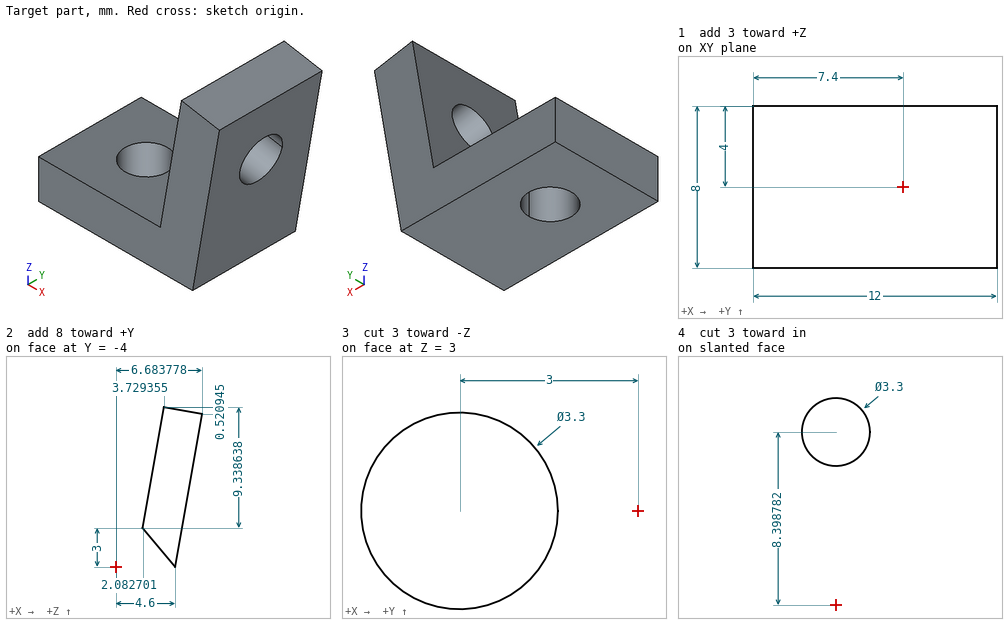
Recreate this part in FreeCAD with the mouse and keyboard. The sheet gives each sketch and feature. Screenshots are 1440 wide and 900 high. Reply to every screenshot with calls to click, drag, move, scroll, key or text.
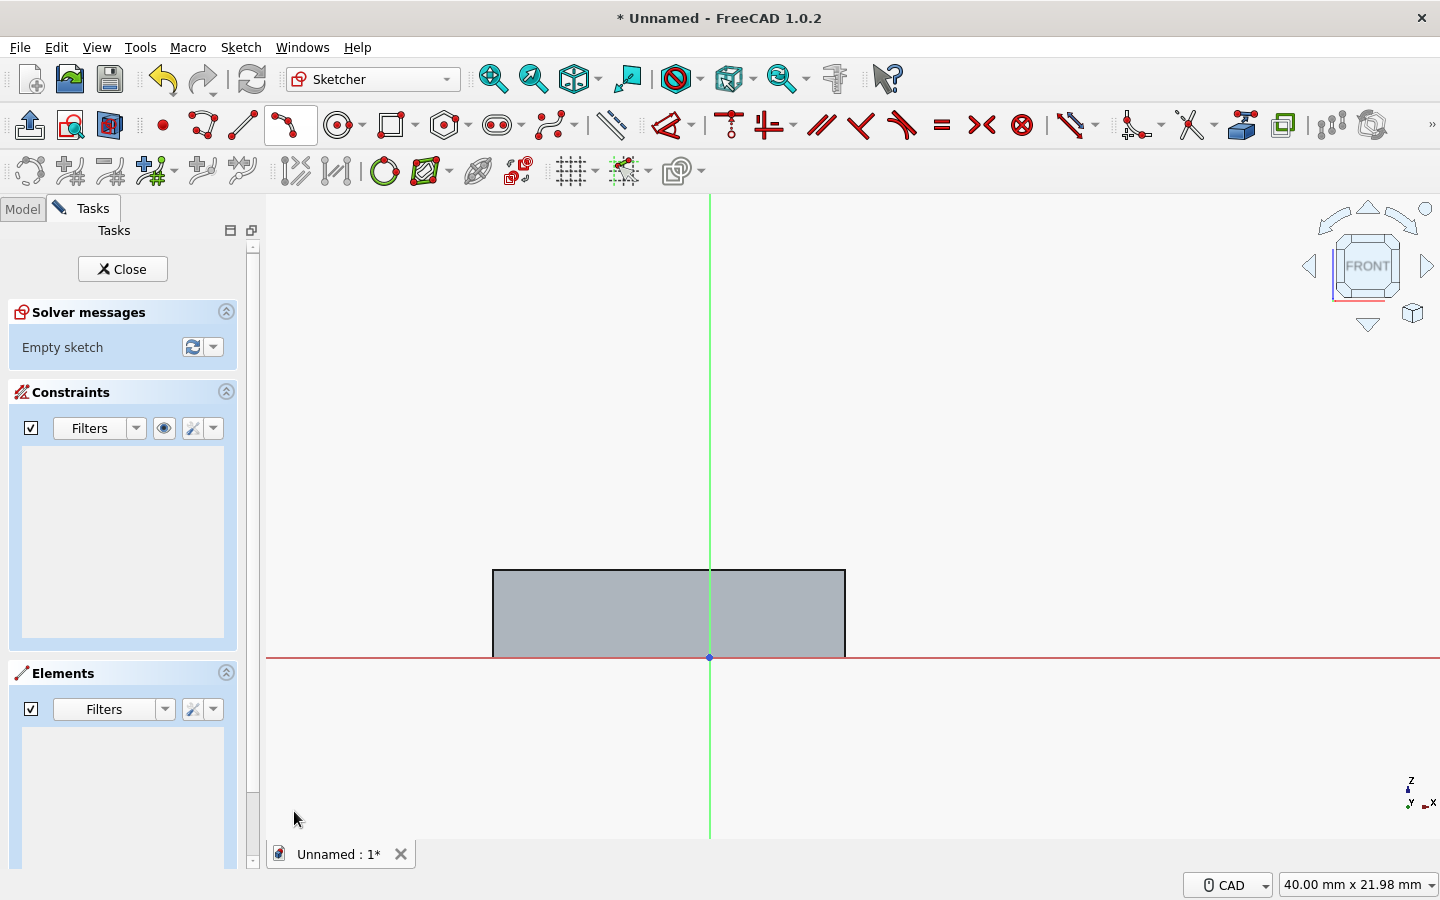
key(g)
key(m)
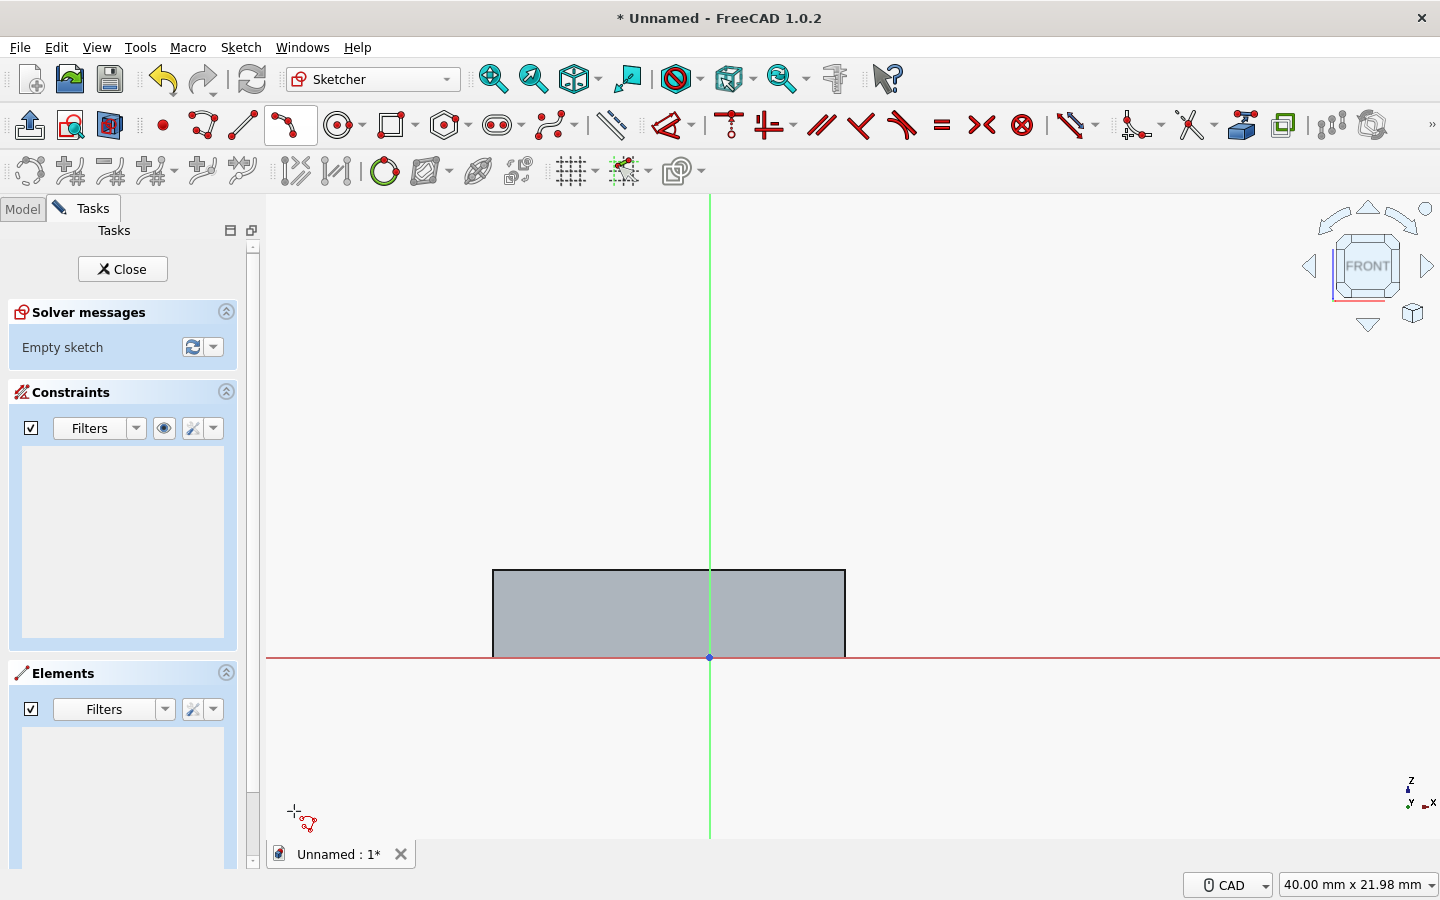
click(771, 570)
click(845, 658)
click(906, 311)
click(819, 296)
click(771, 571)
key(Escape)
key(Escape)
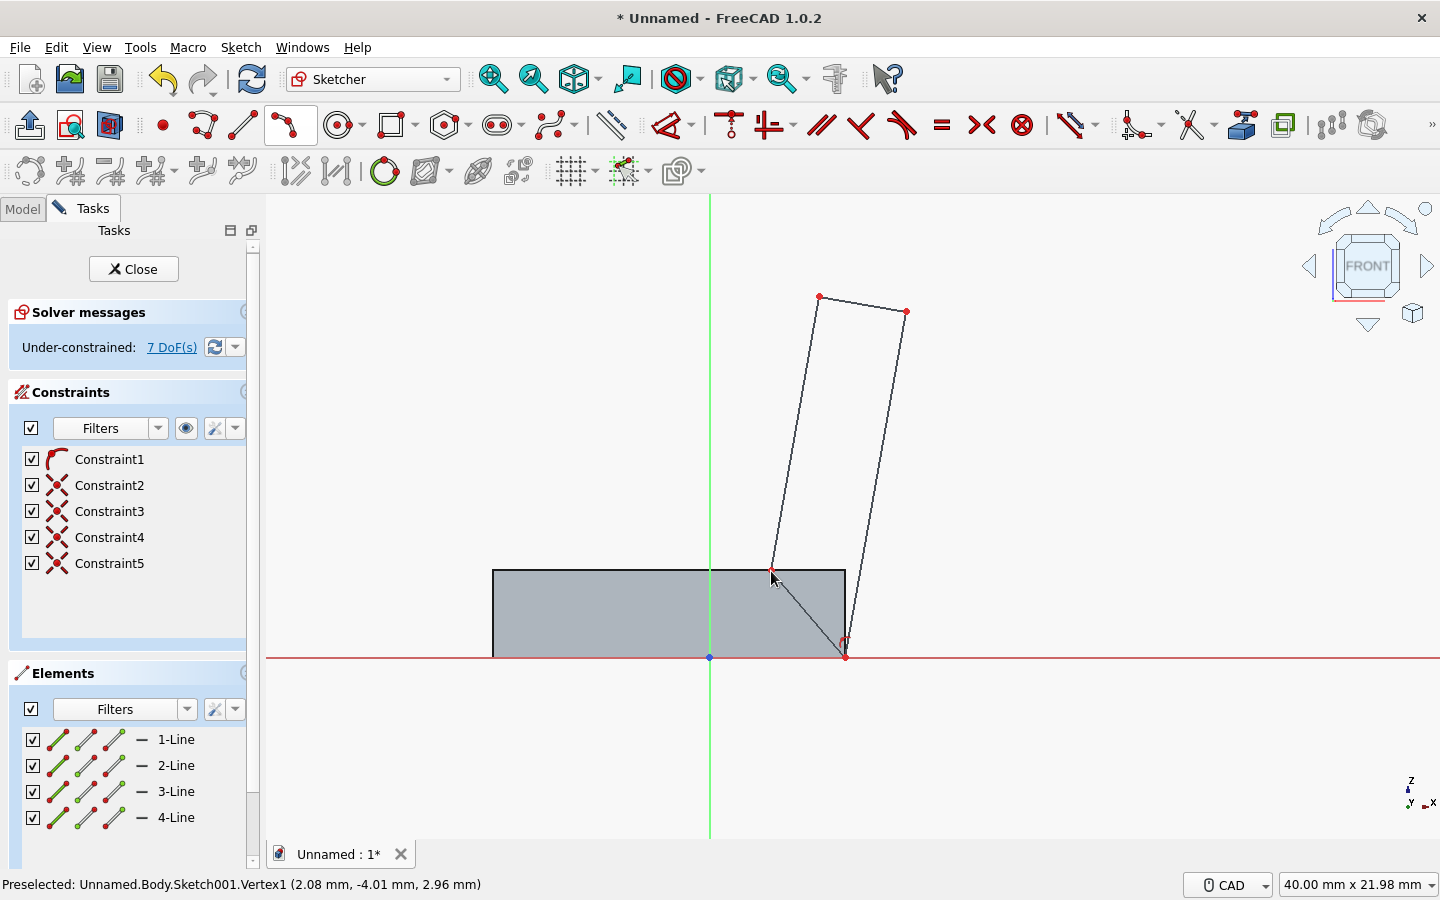
click(666, 126)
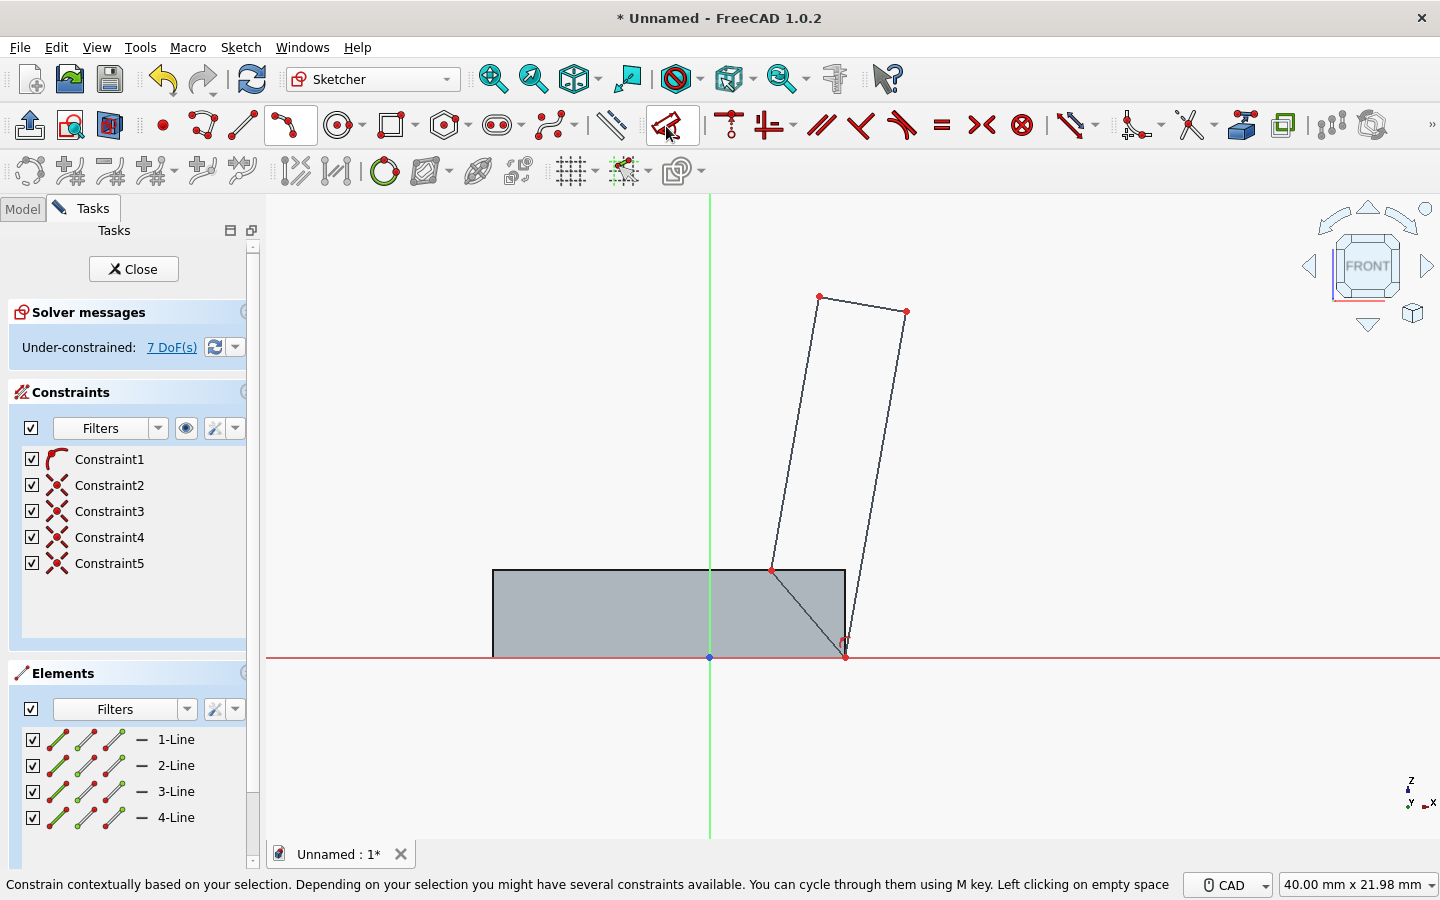
click(771, 571)
click(676, 614)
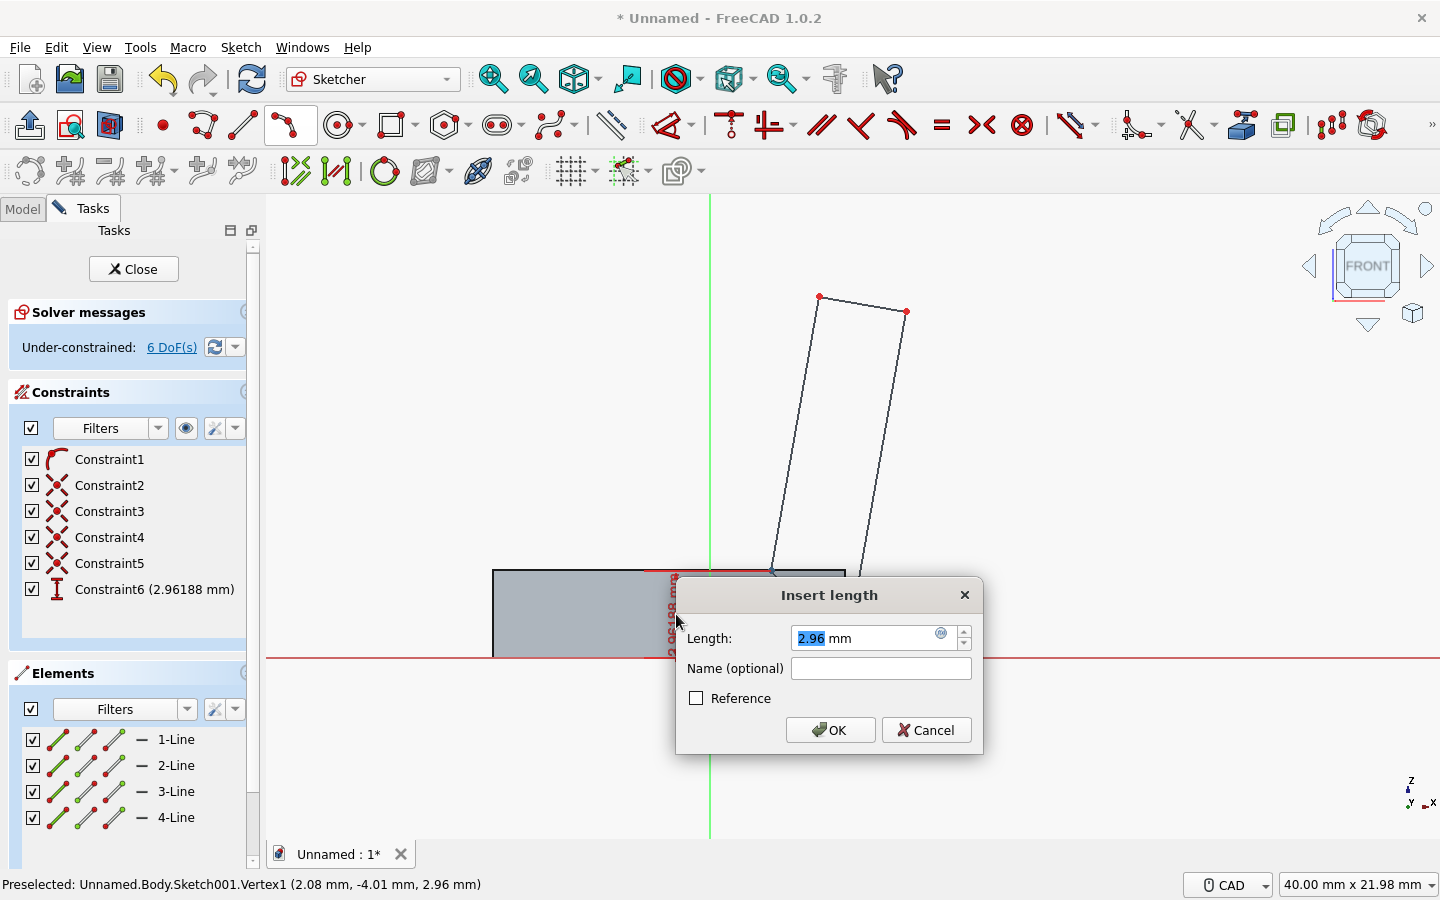
text(3)
key(Return)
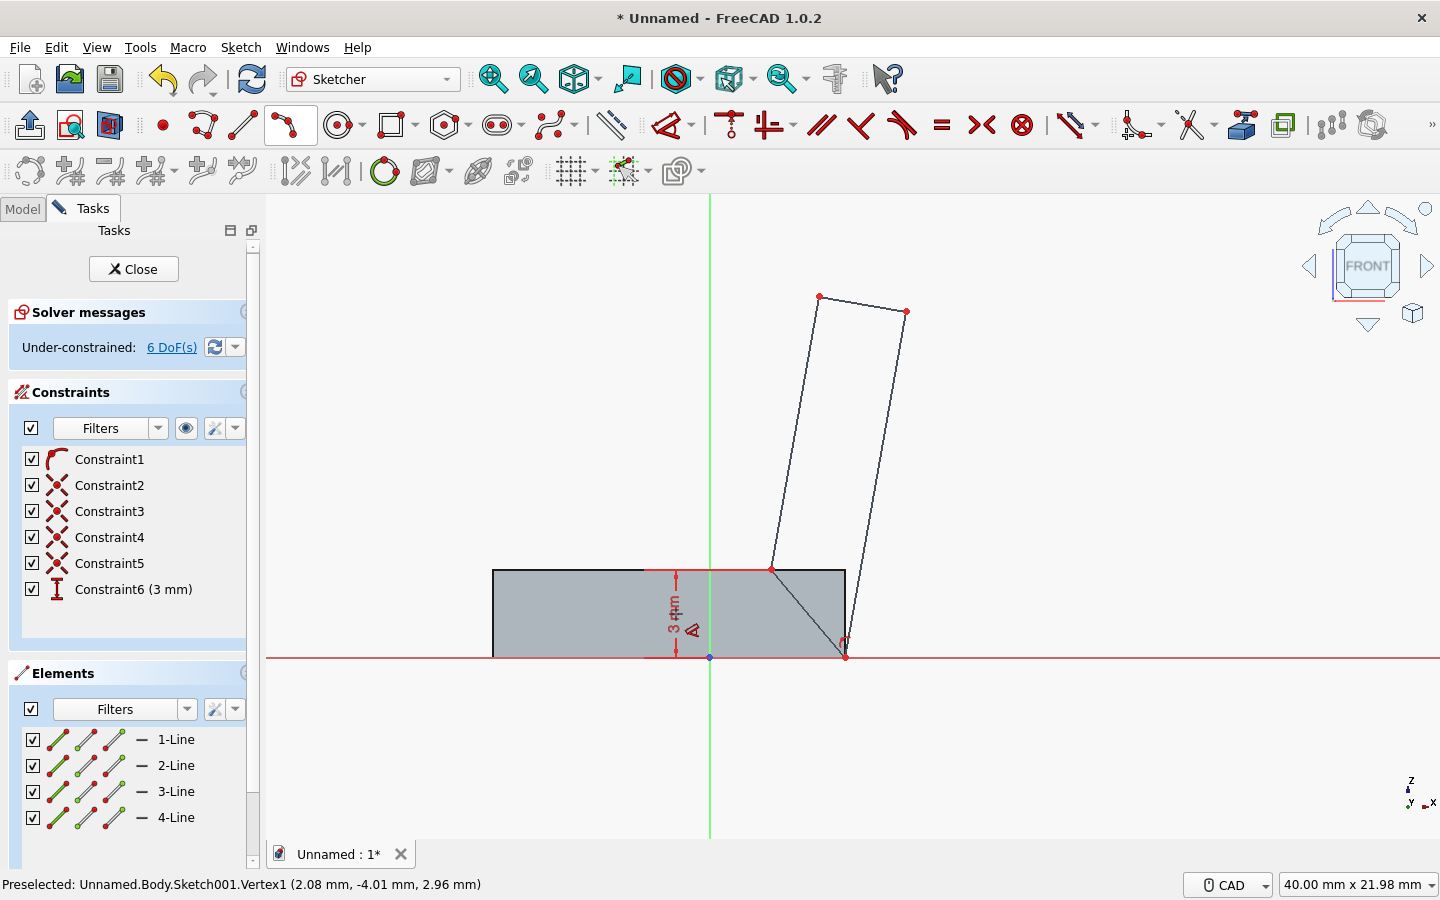
click(845, 658)
click(777, 692)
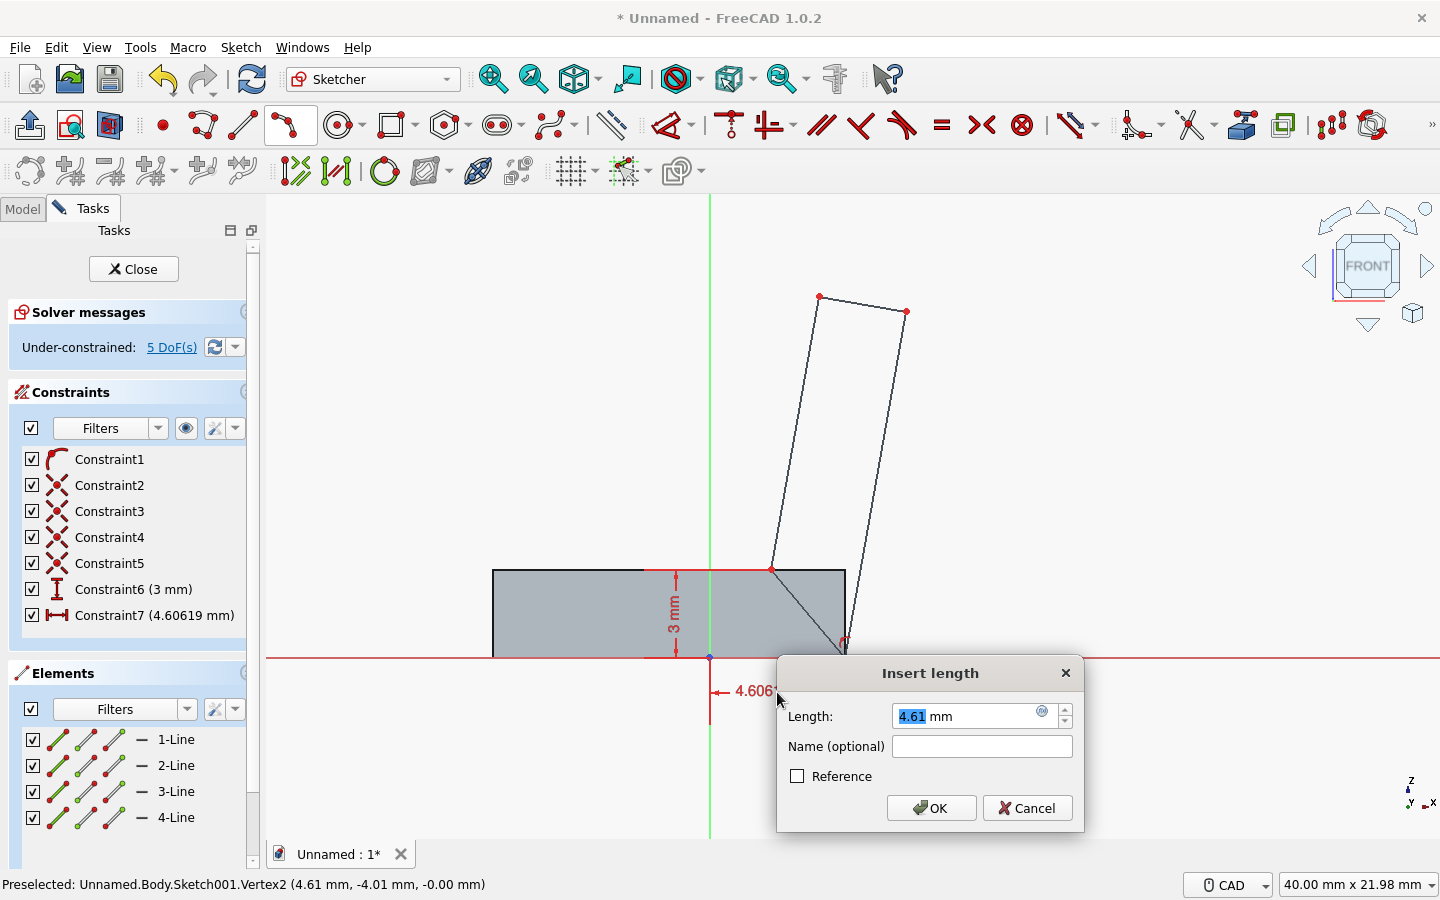
text(4.6)
key(Return)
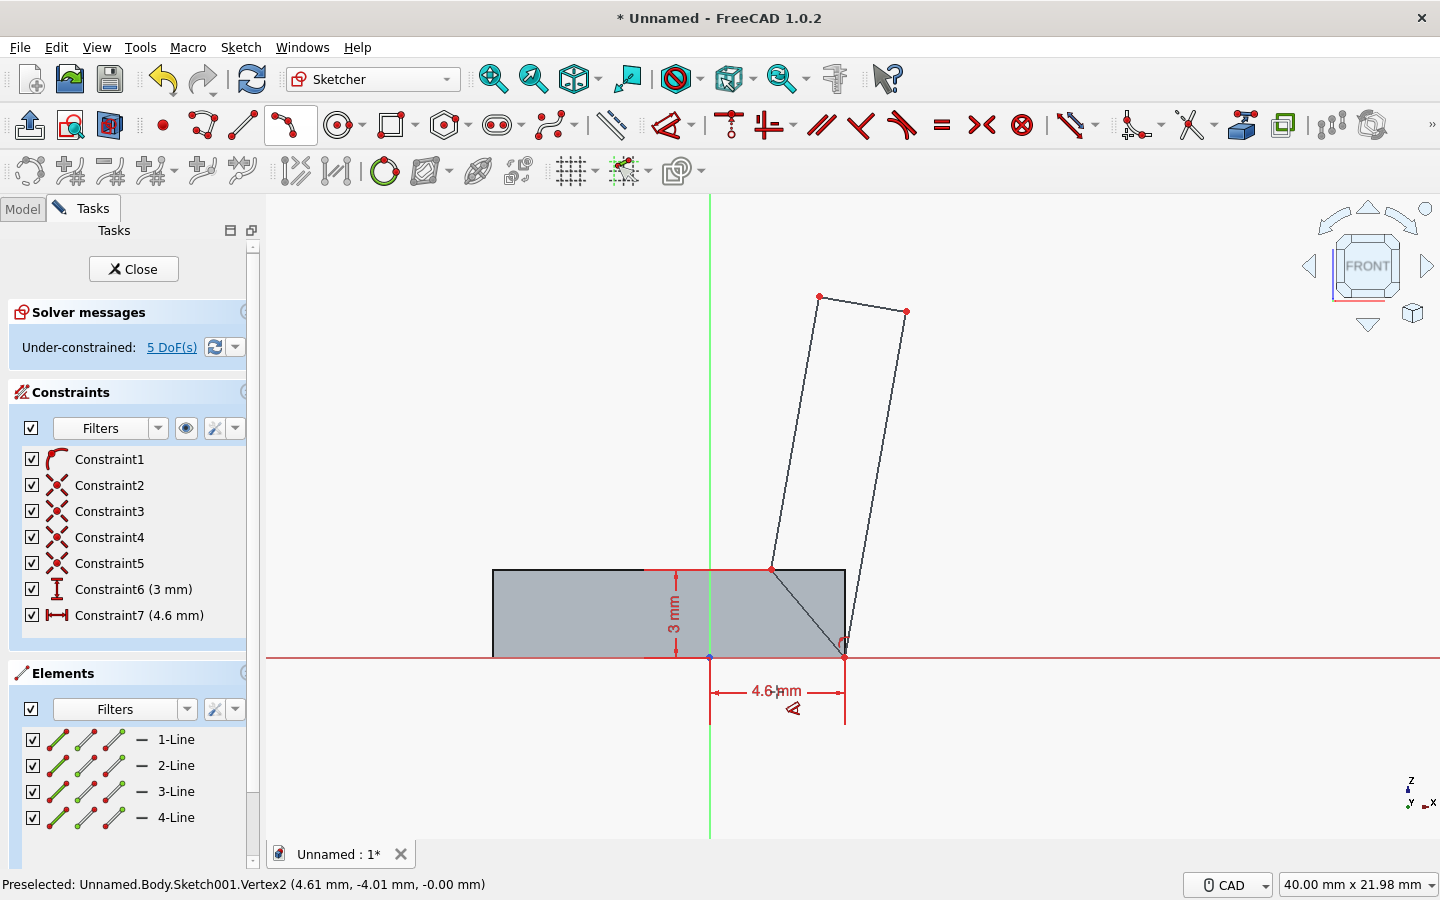
click(771, 570)
click(740, 536)